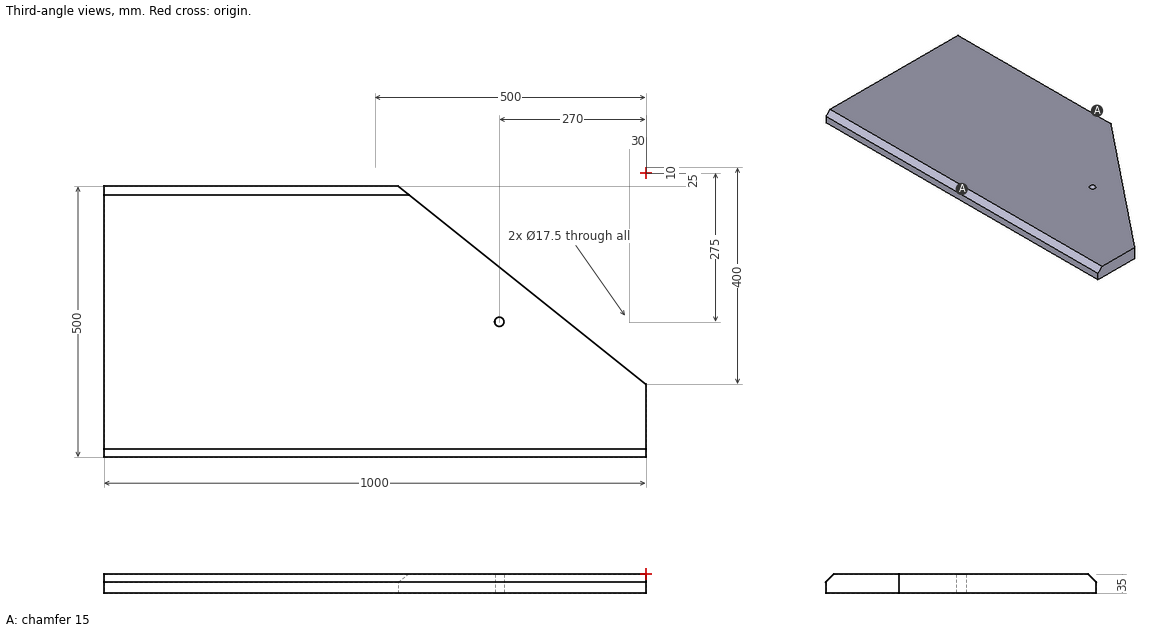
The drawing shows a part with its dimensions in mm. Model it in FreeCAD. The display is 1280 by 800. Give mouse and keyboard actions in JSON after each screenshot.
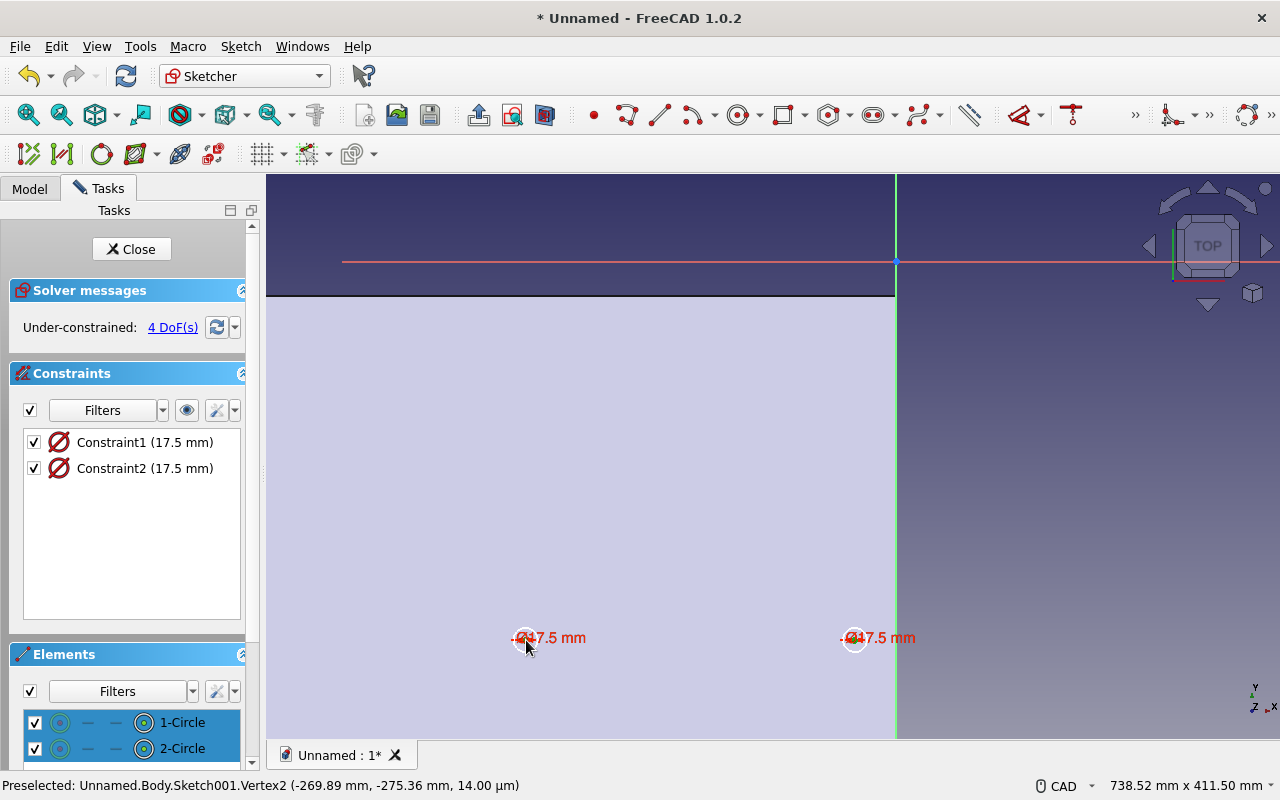
{"action": "key", "text": "h"}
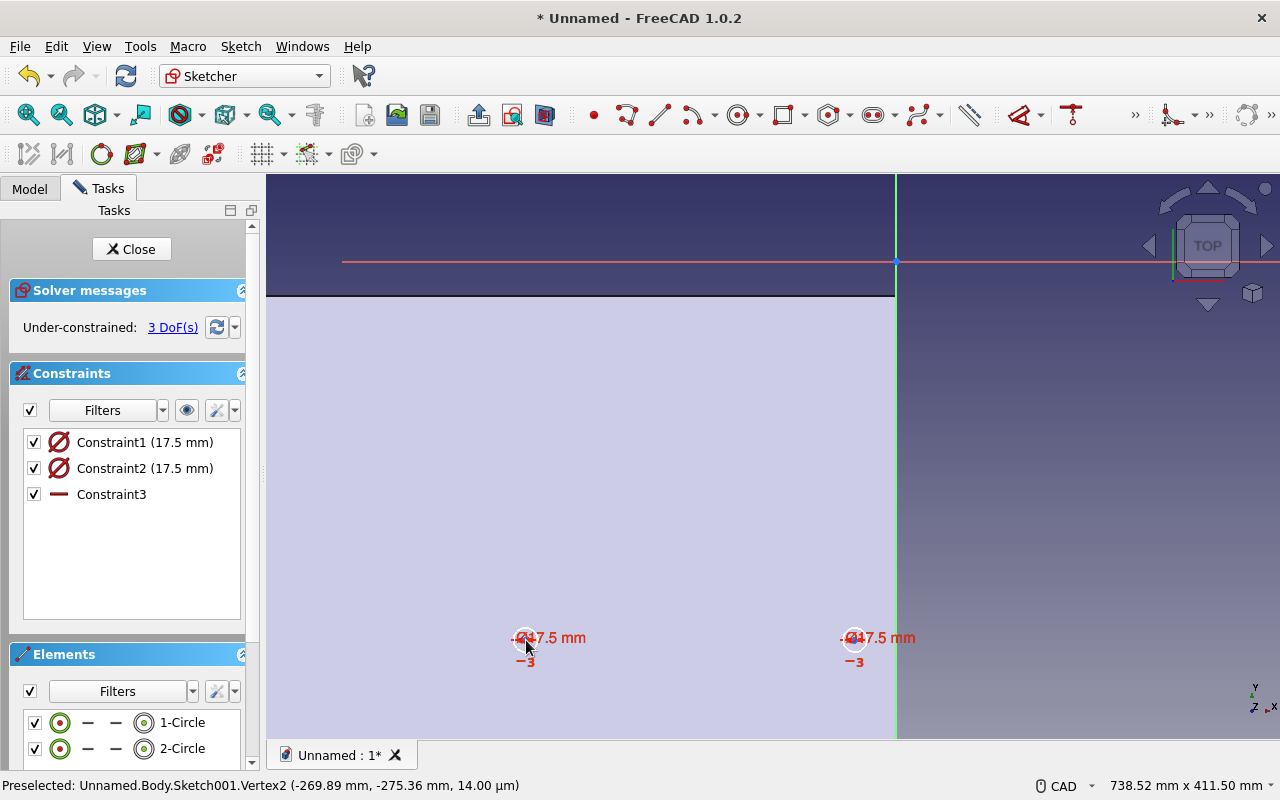
{"action": "key", "text": "d"}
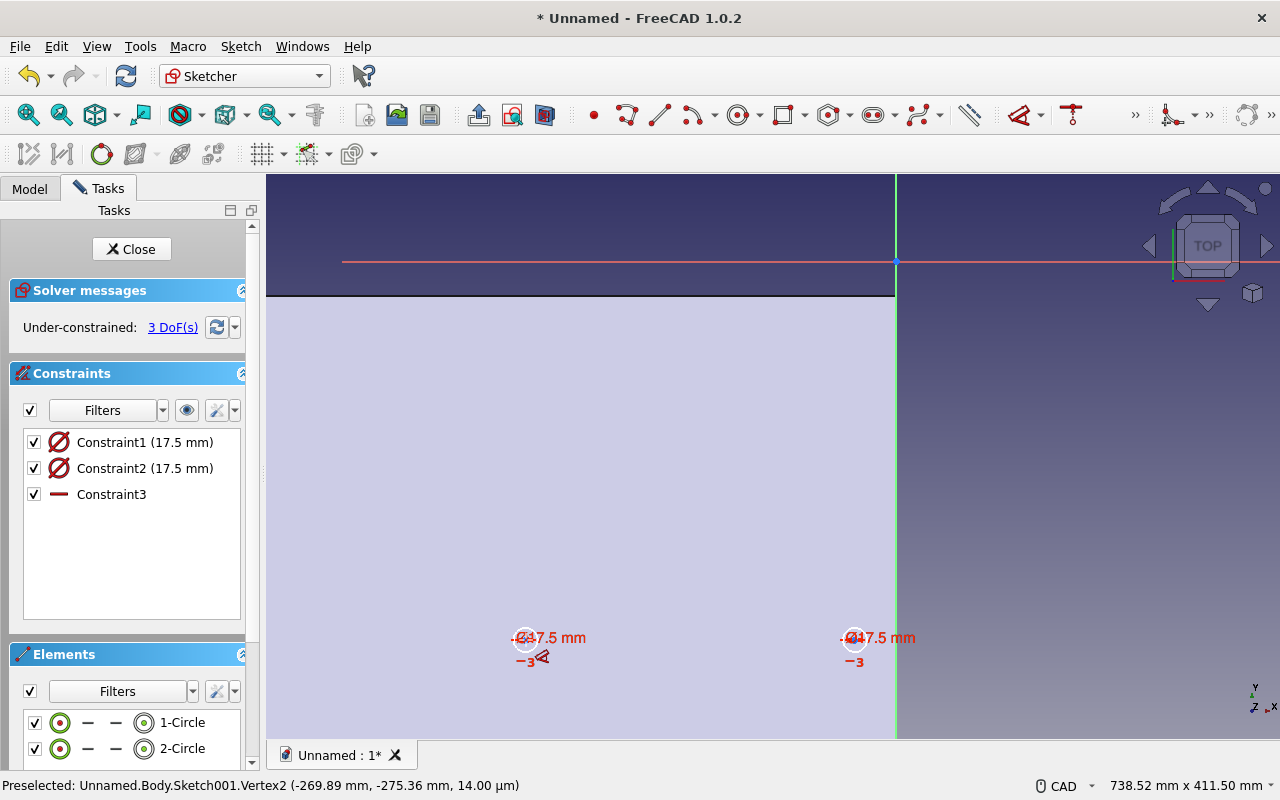
{"action": "left_click", "coordinate": [855, 640]}
{"action": "left_click", "coordinate": [876, 228]}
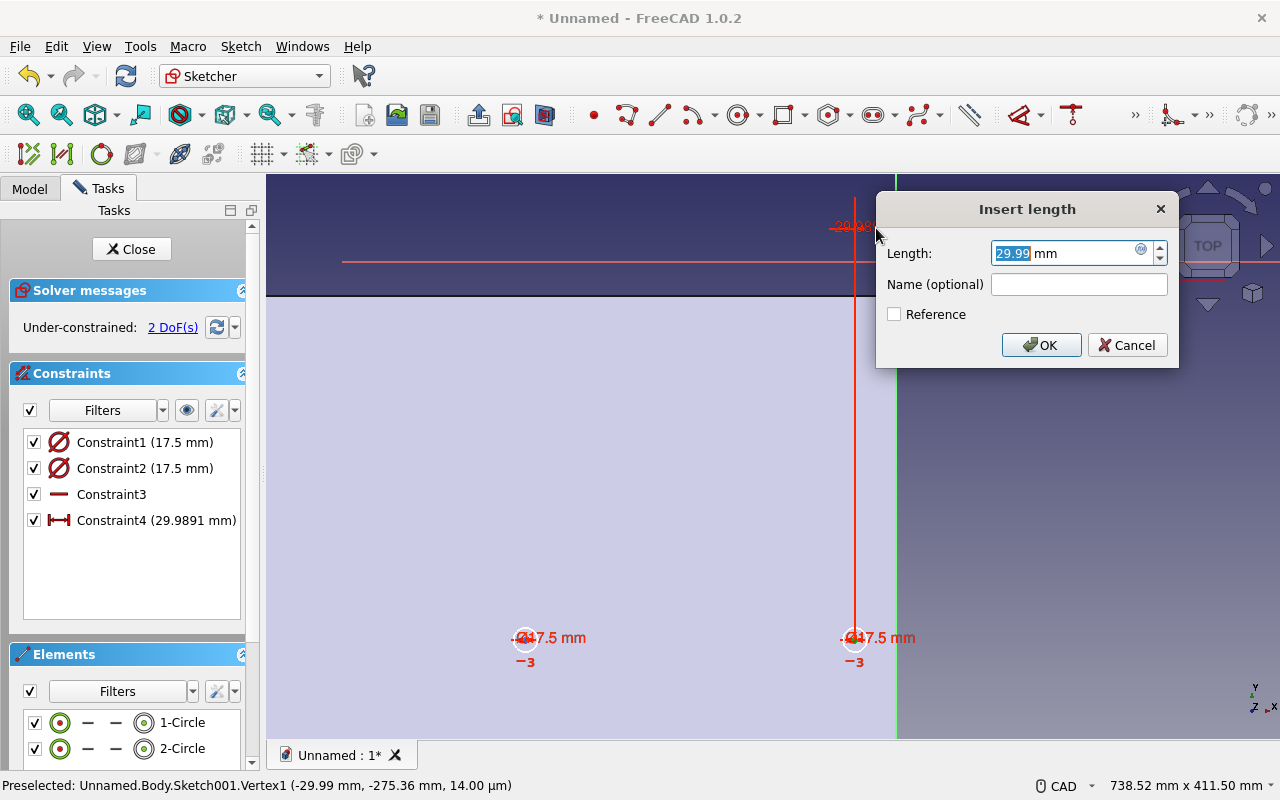
{"action": "type", "text": "30"}
{"action": "key", "text": "Return"}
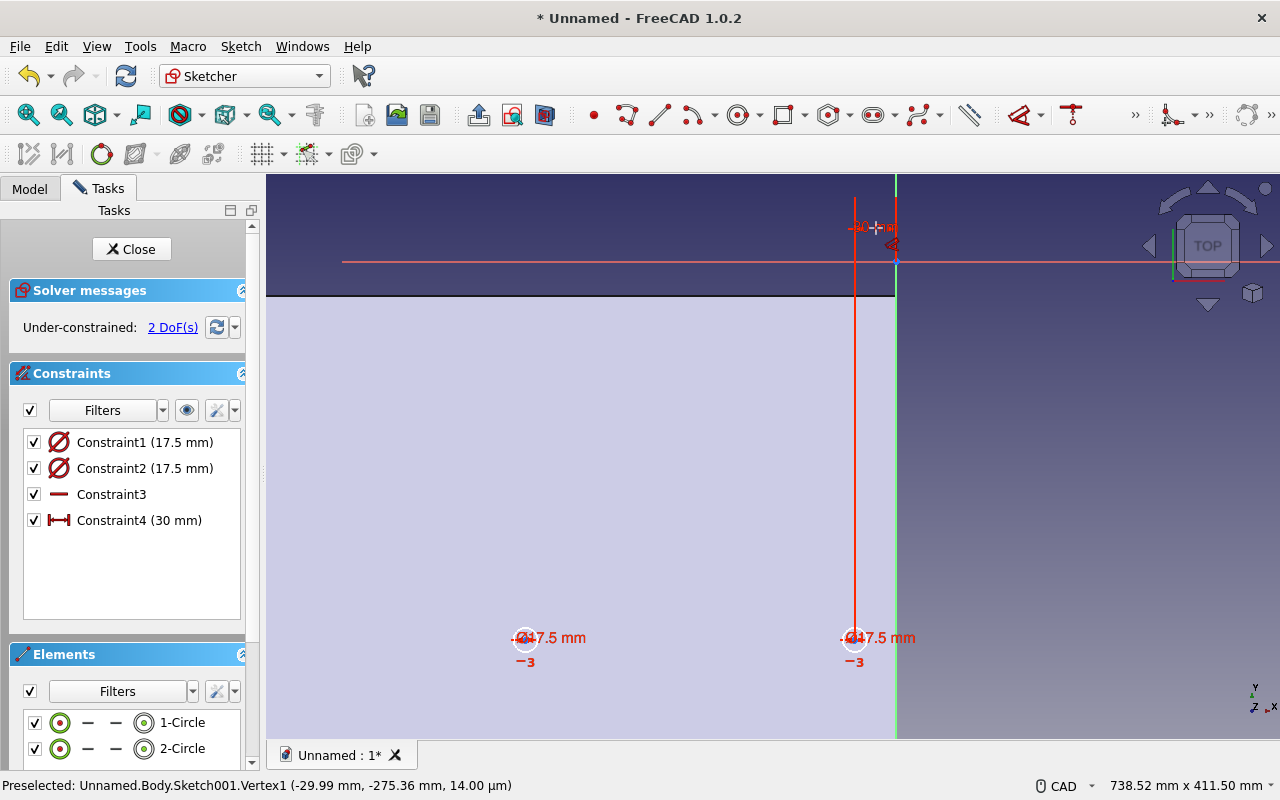
{"action": "left_click", "coordinate": [855, 640]}
{"action": "left_click", "coordinate": [930, 451]}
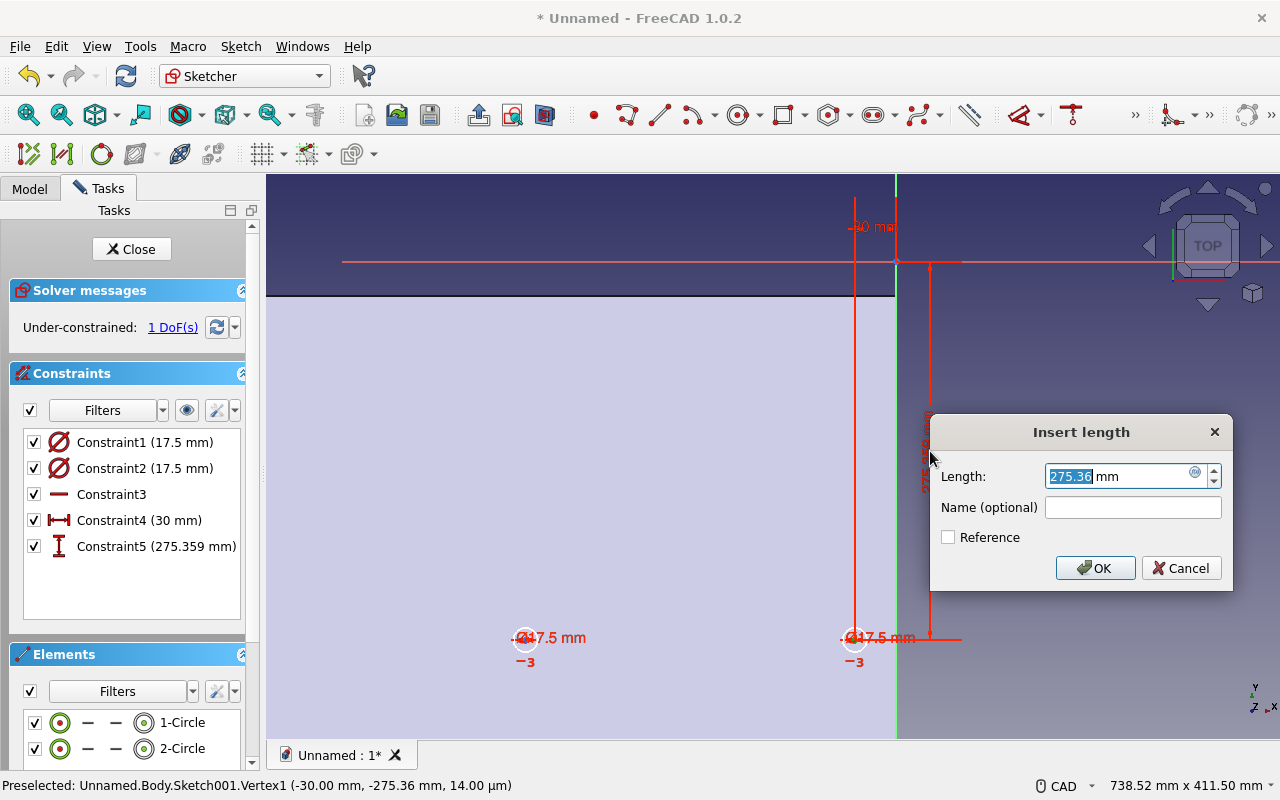
{"action": "type", "text": "275"}
{"action": "key", "text": "Return"}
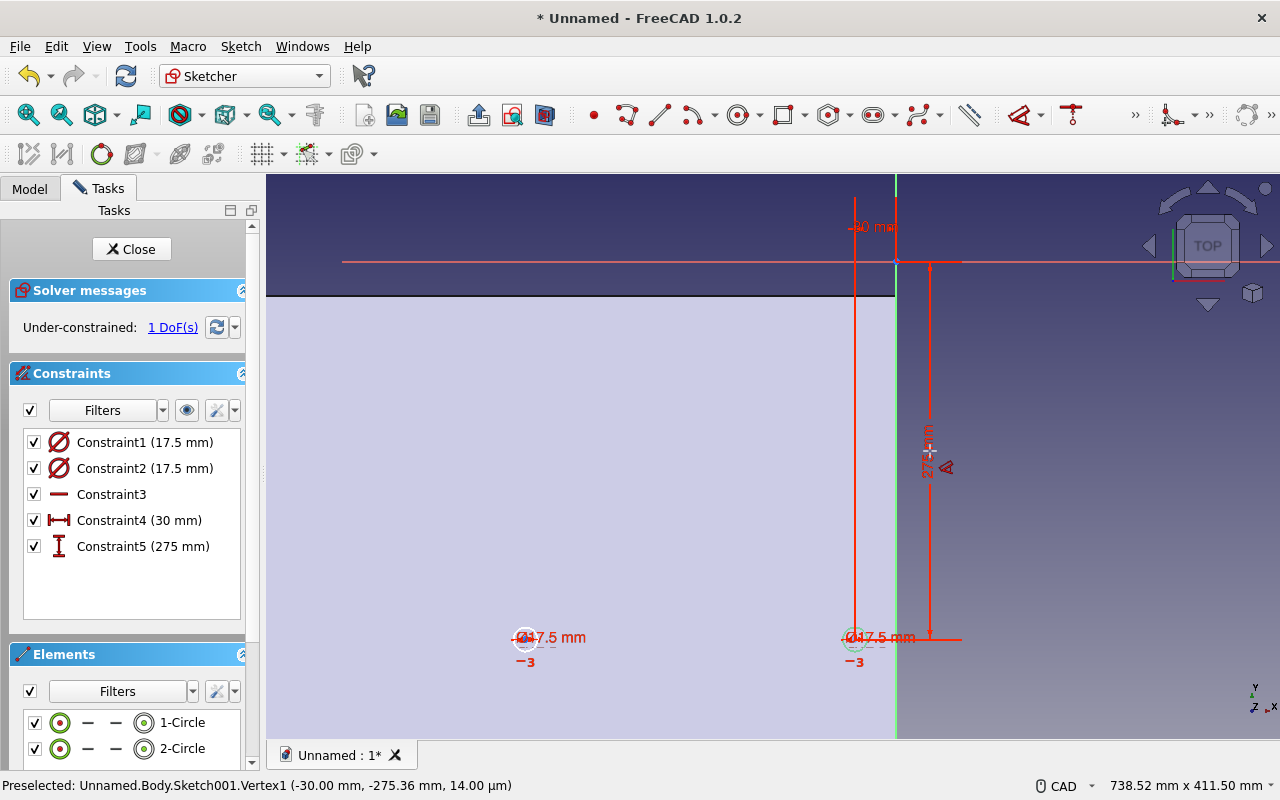
{"action": "left_click", "coordinate": [526, 640]}
{"action": "left_click", "coordinate": [711, 228]}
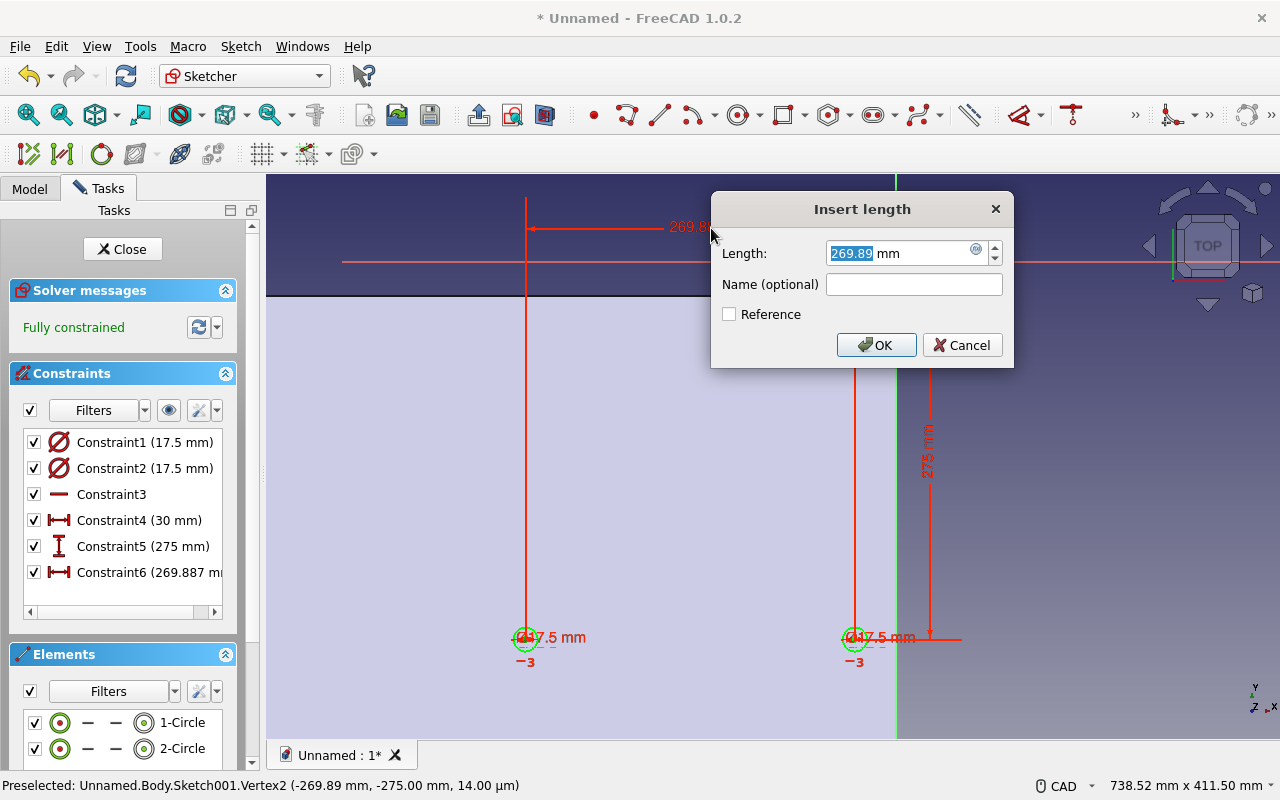
{"action": "type", "text": "270"}
{"action": "key", "text": "Return"}
{"action": "key", "text": "Escape"}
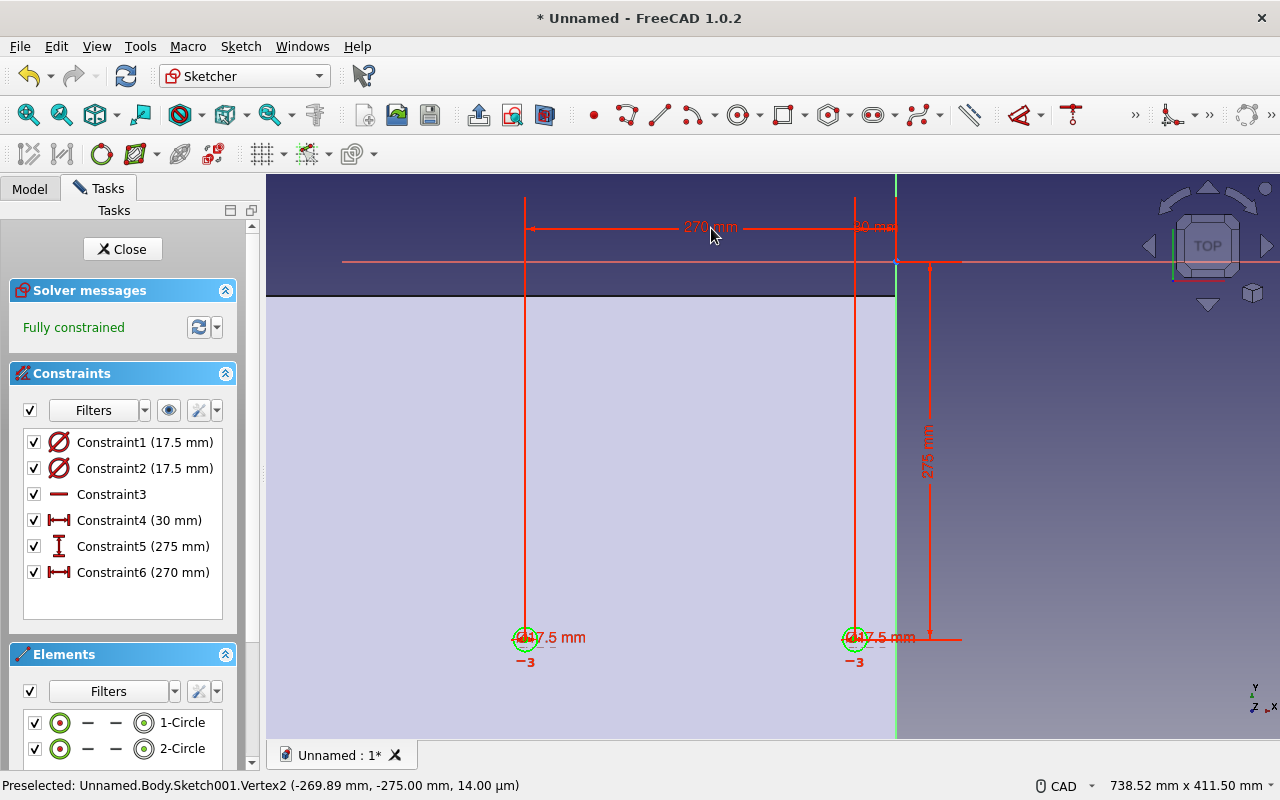
{"action": "left_click", "coordinate": [123, 249]}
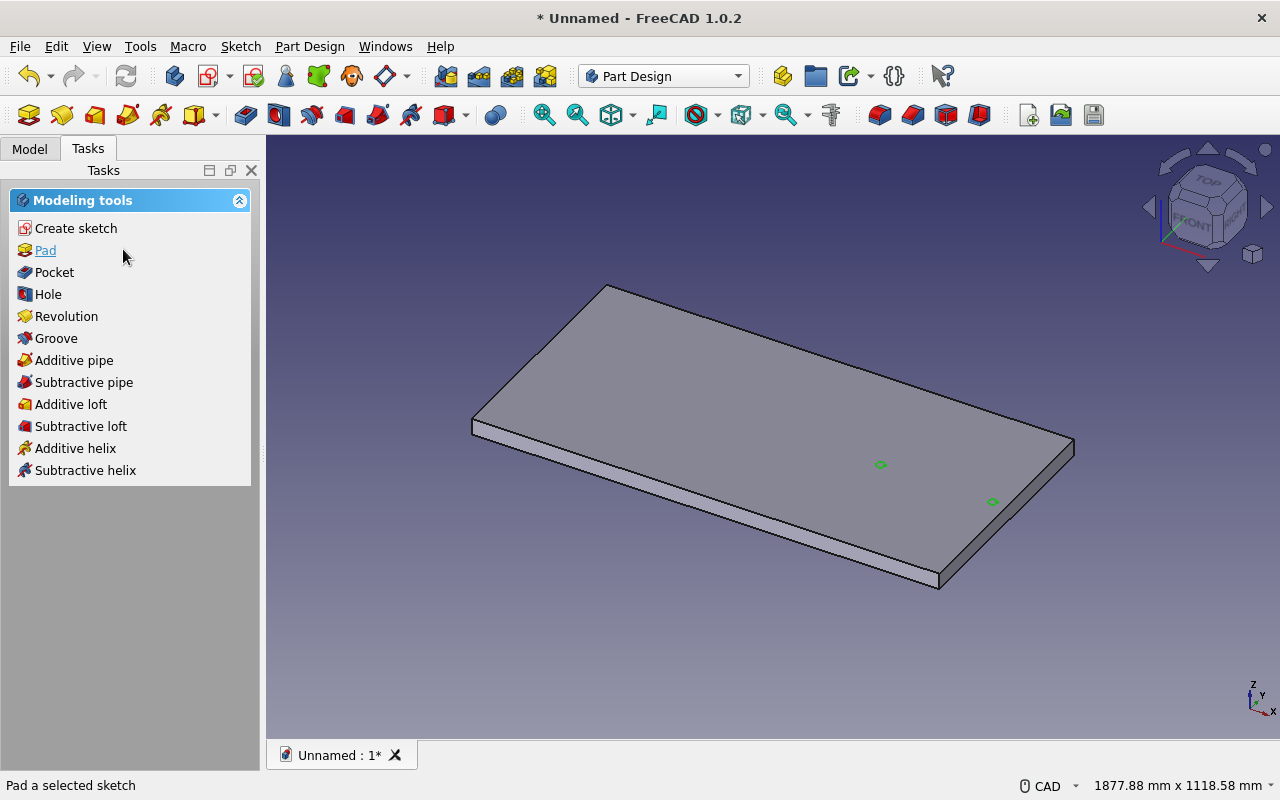
{"action": "left_click", "coordinate": [279, 116]}